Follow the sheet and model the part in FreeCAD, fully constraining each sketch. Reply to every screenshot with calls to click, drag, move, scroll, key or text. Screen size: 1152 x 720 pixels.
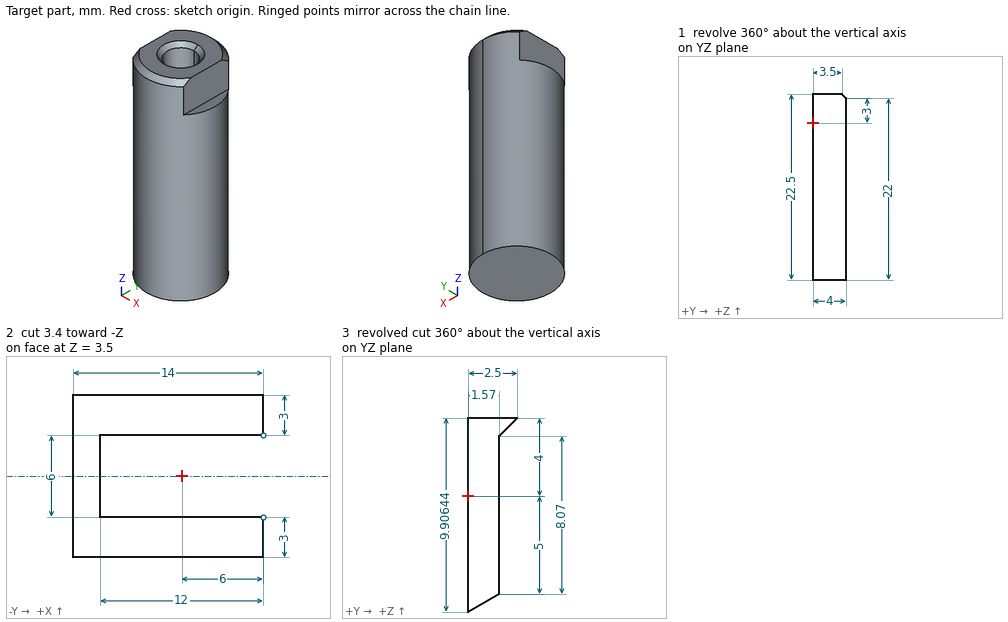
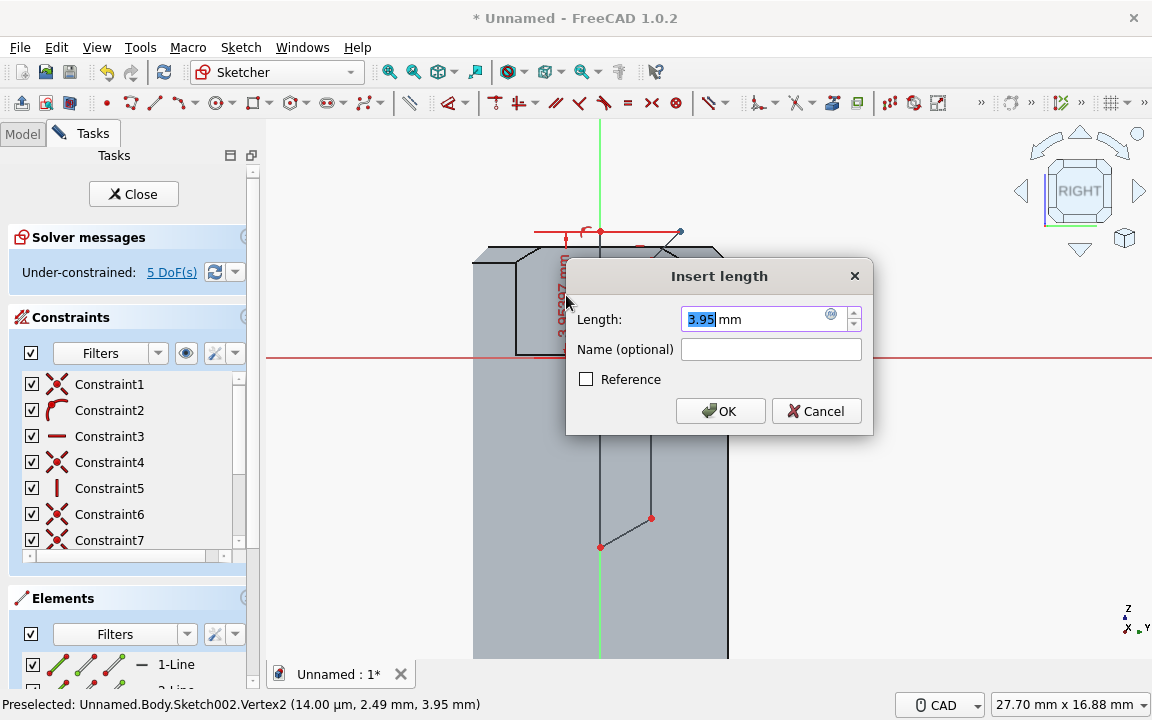
text(4)
key(Return)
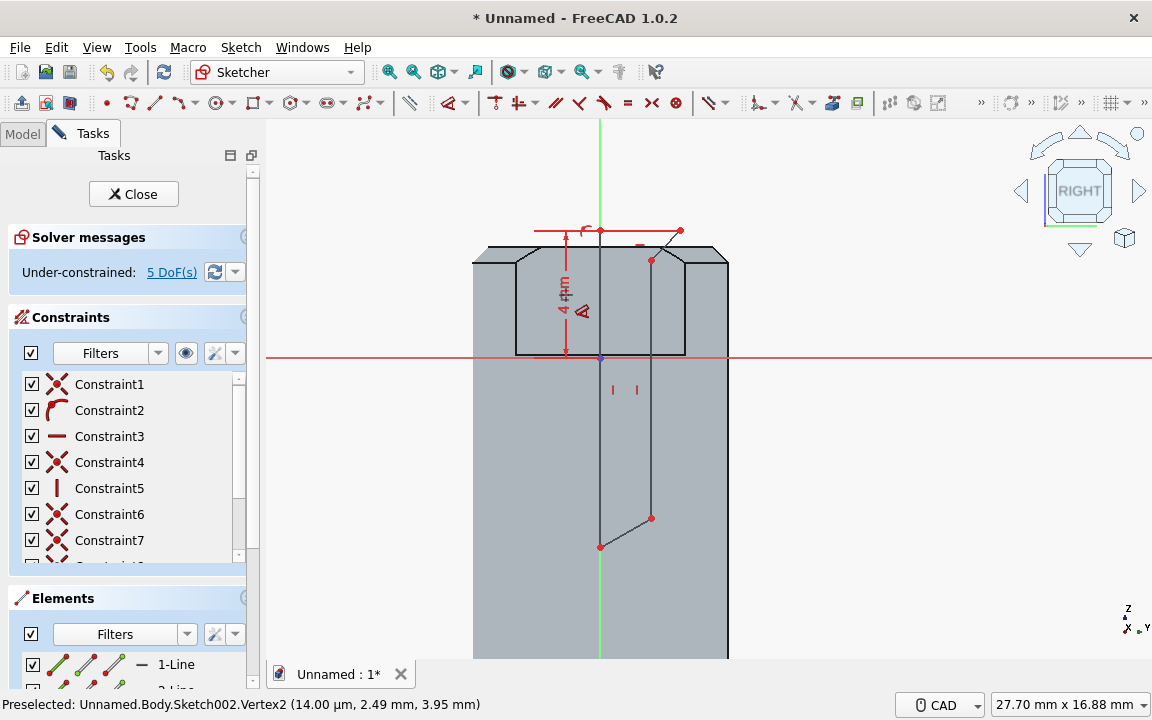
click(651, 519)
click(566, 439)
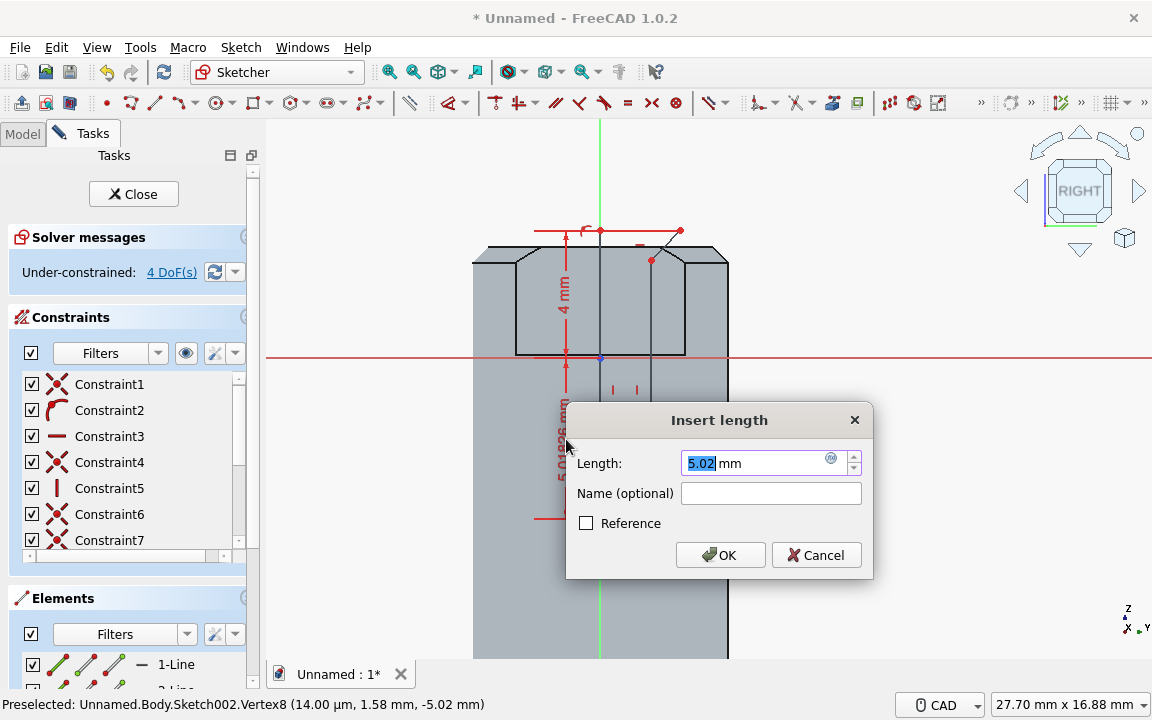
text(5)
key(Return)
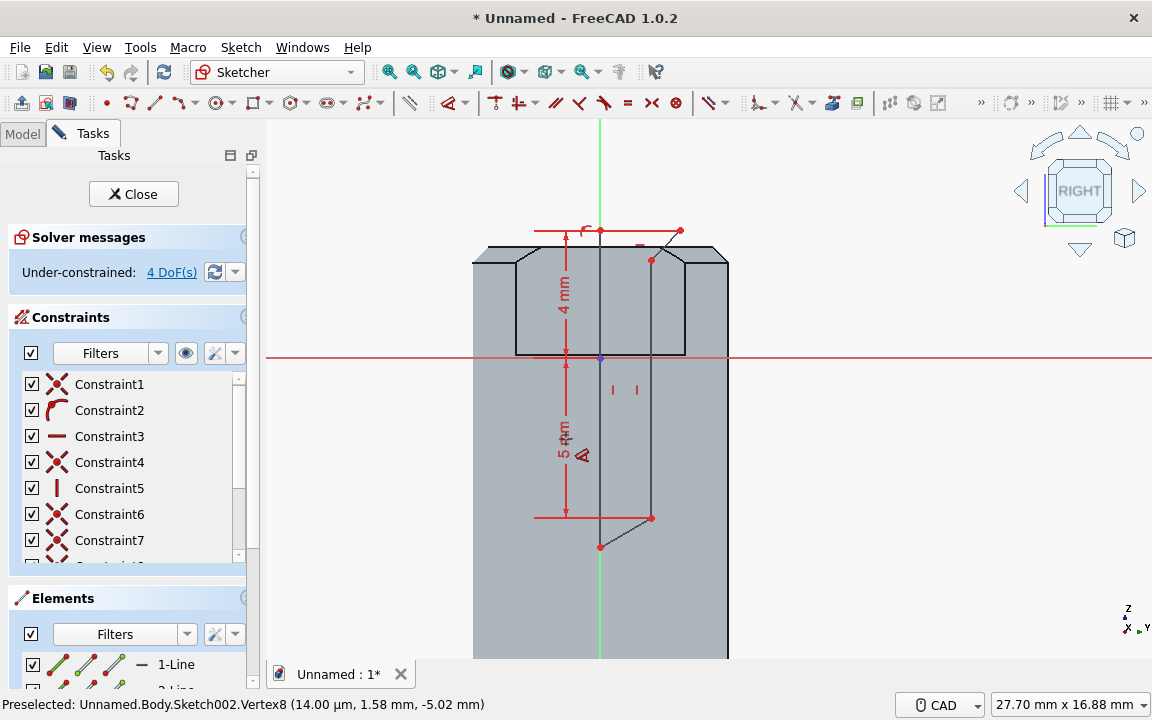
click(656, 231)
click(640, 197)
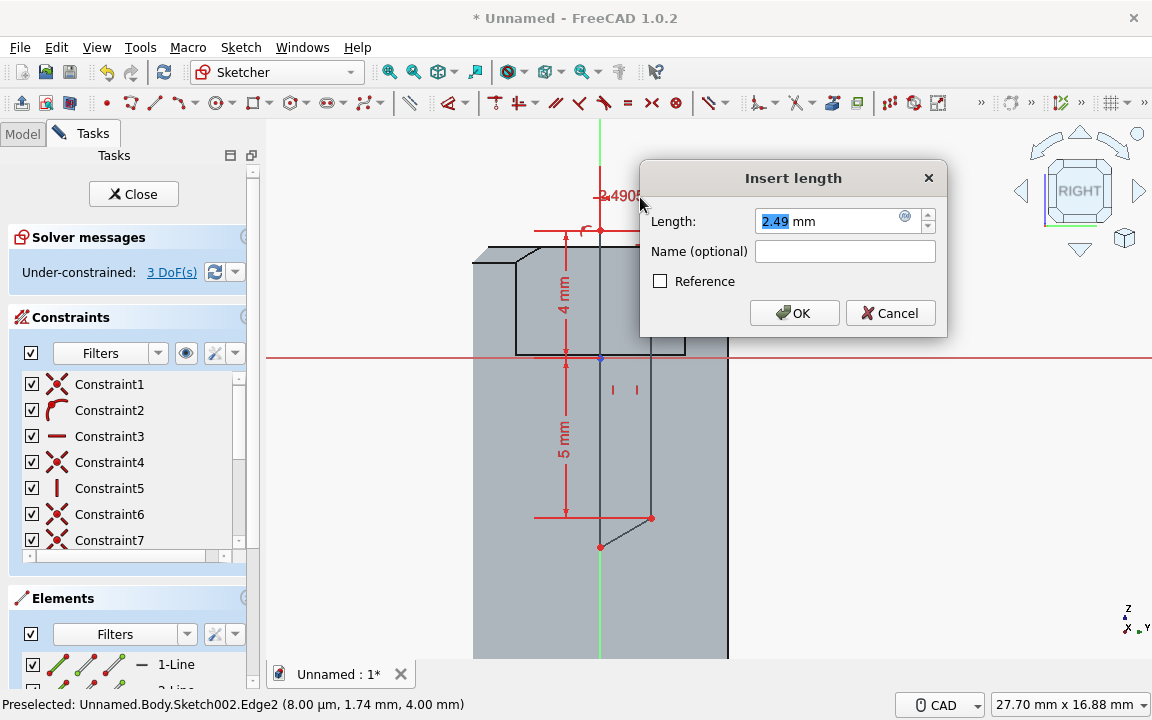
text(2.5)
key(Return)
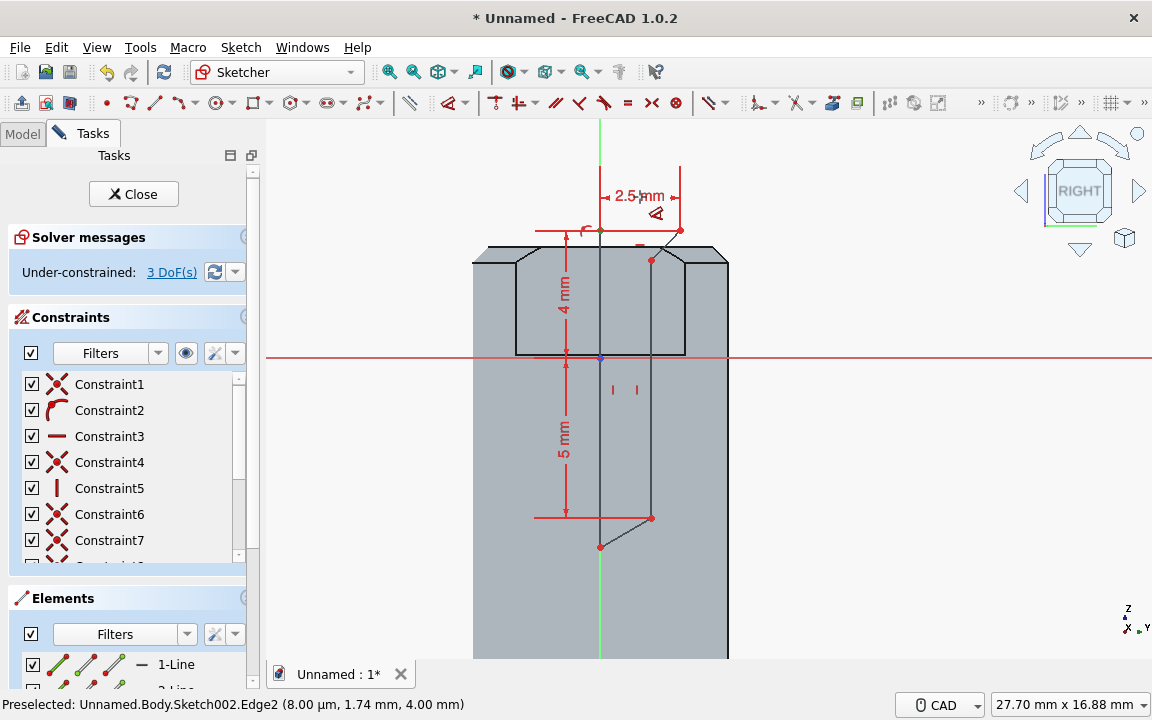
click(651, 441)
click(685, 390)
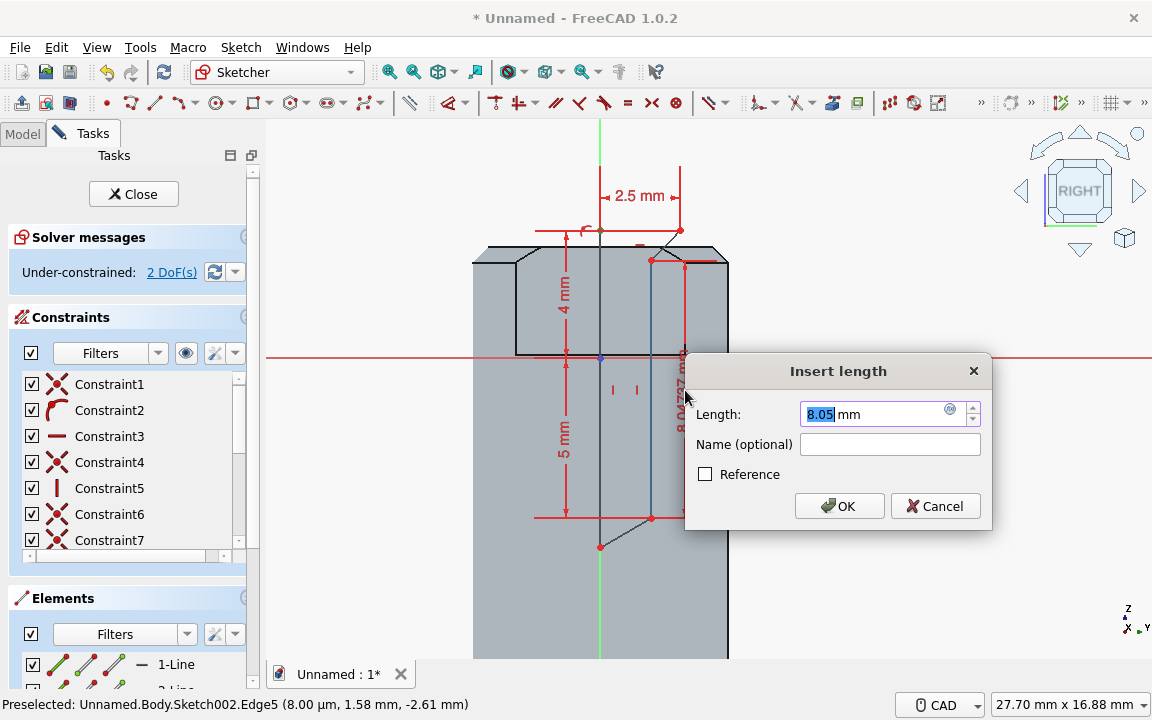
text(8.07)
key(Return)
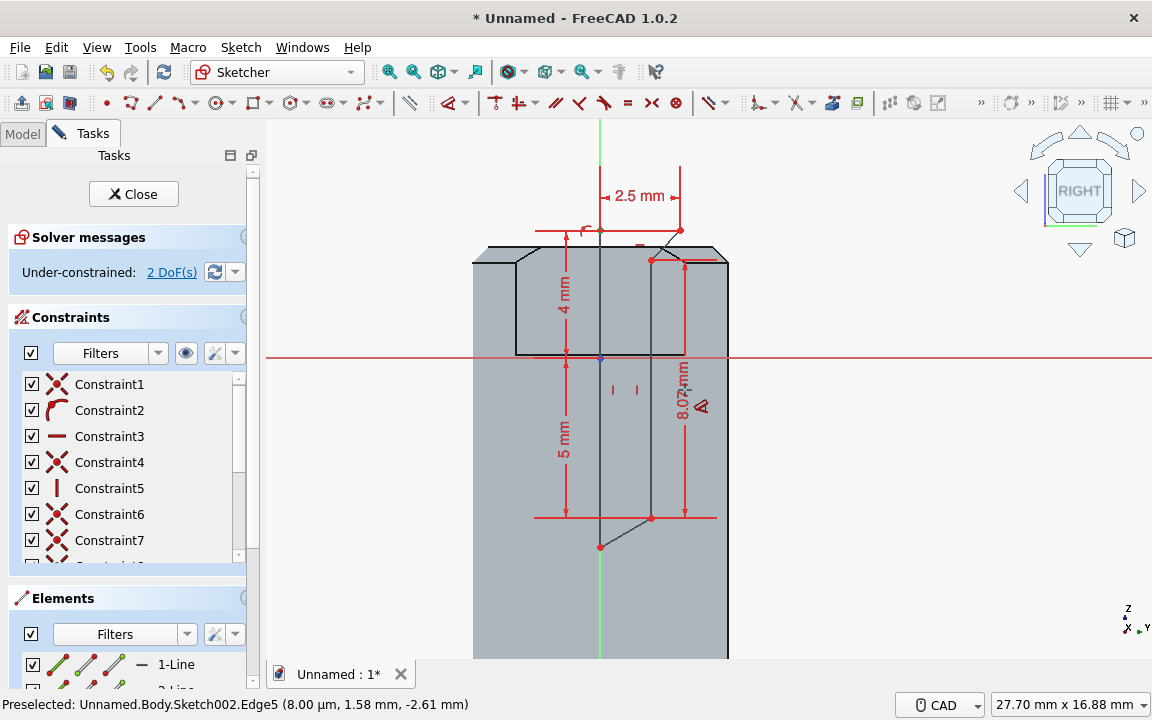
click(651, 260)
click(614, 392)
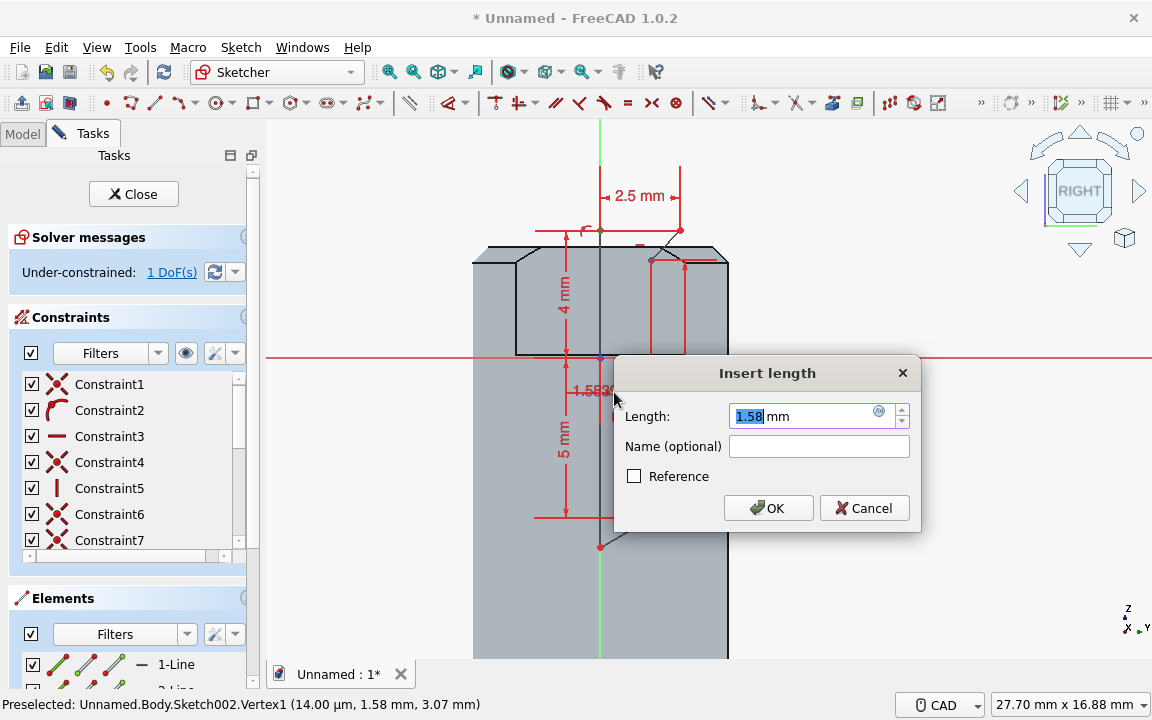
text(1.57)
key(Return)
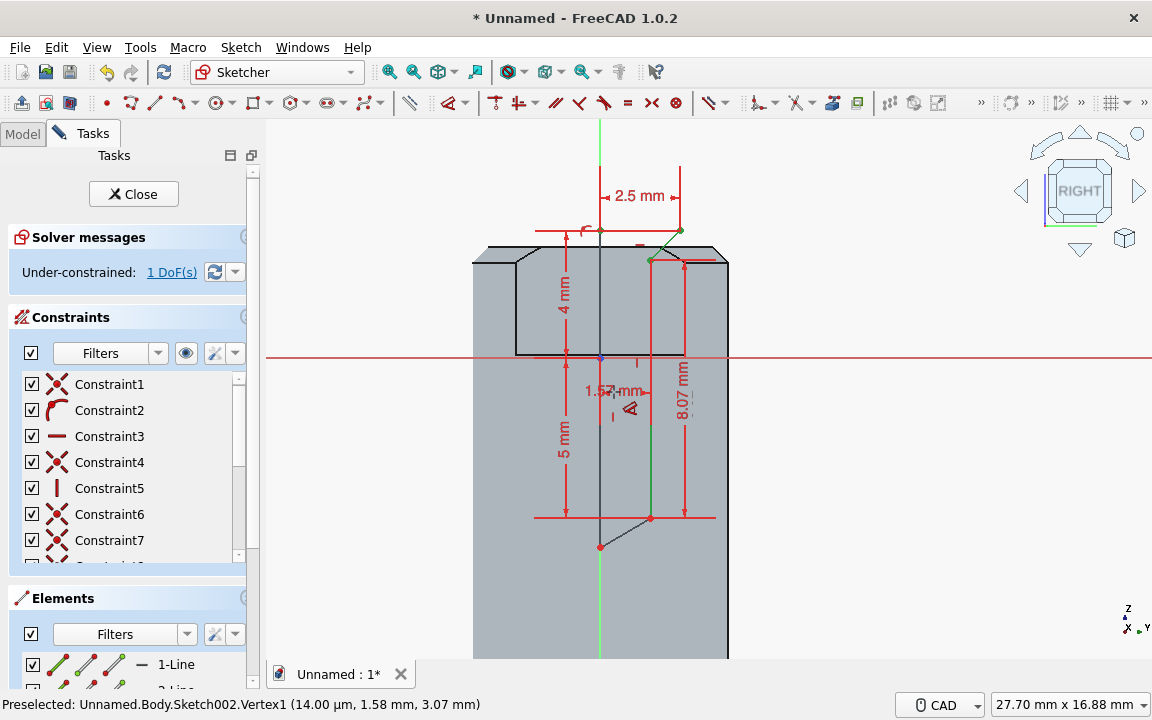
click(600, 326)
click(566, 316)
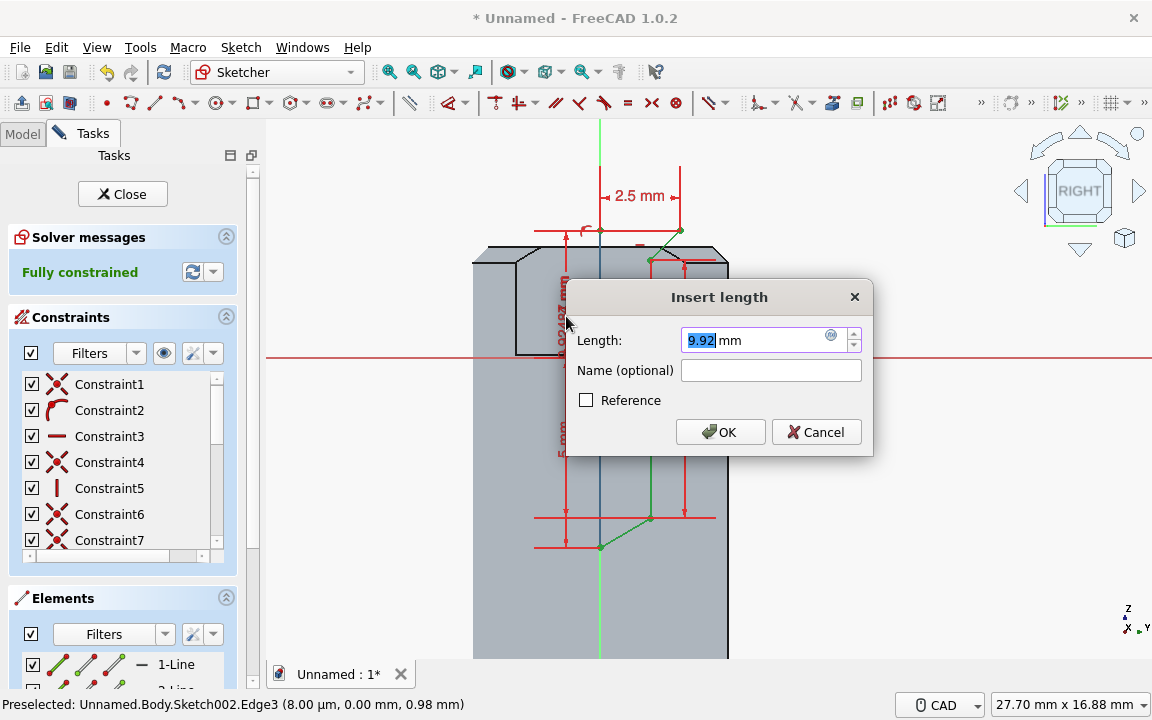
text(9.90644)
key(Return)
key(Escape)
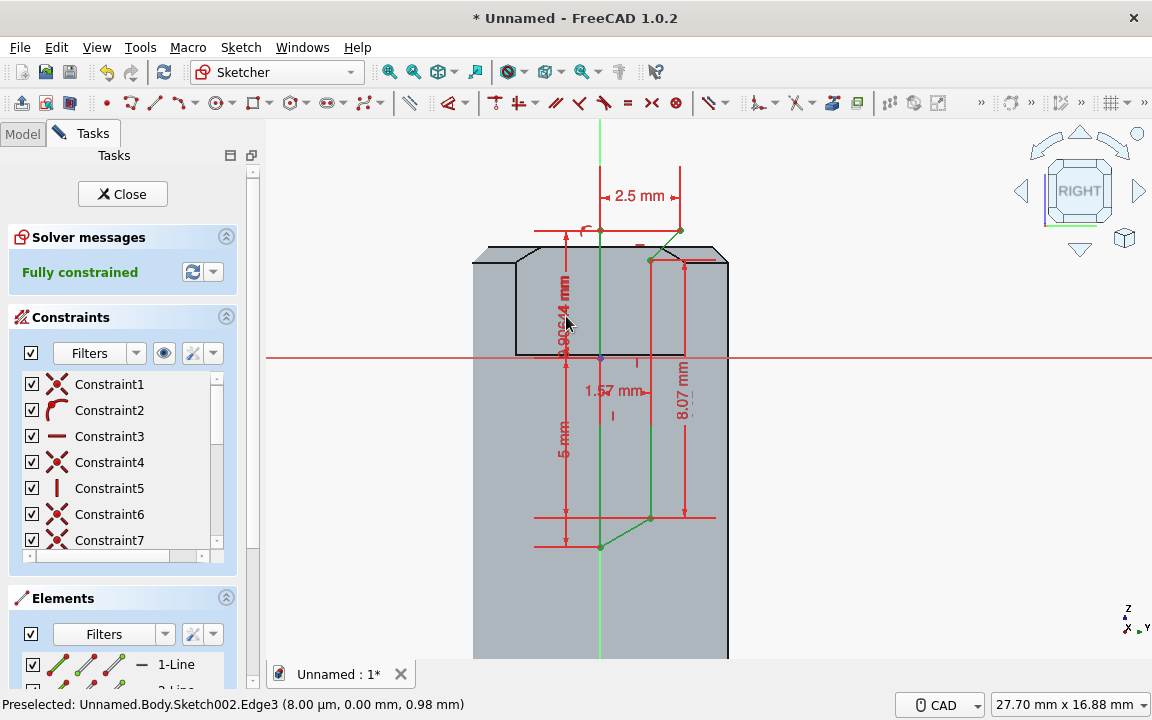
click(123, 194)